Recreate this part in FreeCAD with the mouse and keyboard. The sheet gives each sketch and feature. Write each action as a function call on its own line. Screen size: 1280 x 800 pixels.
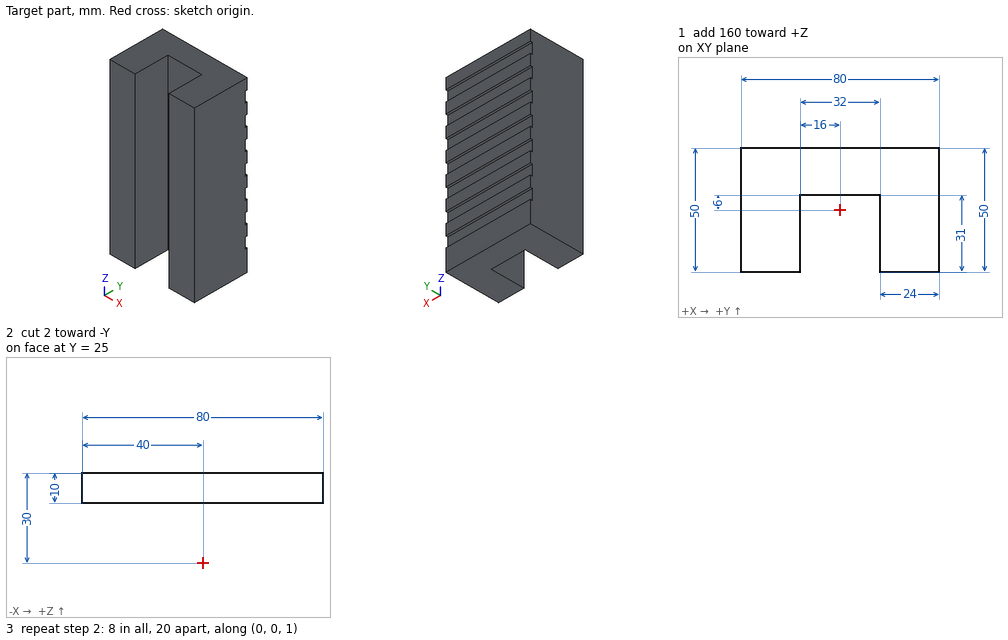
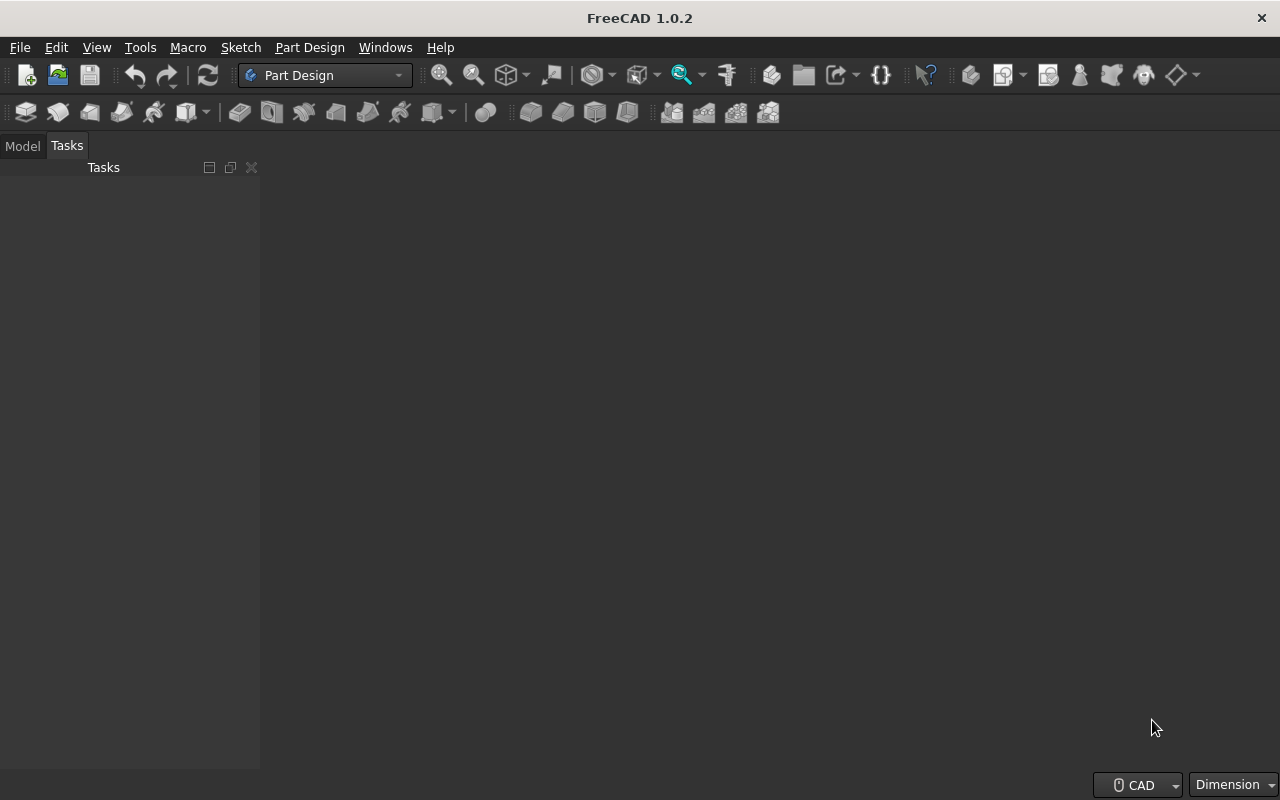
click(26, 76)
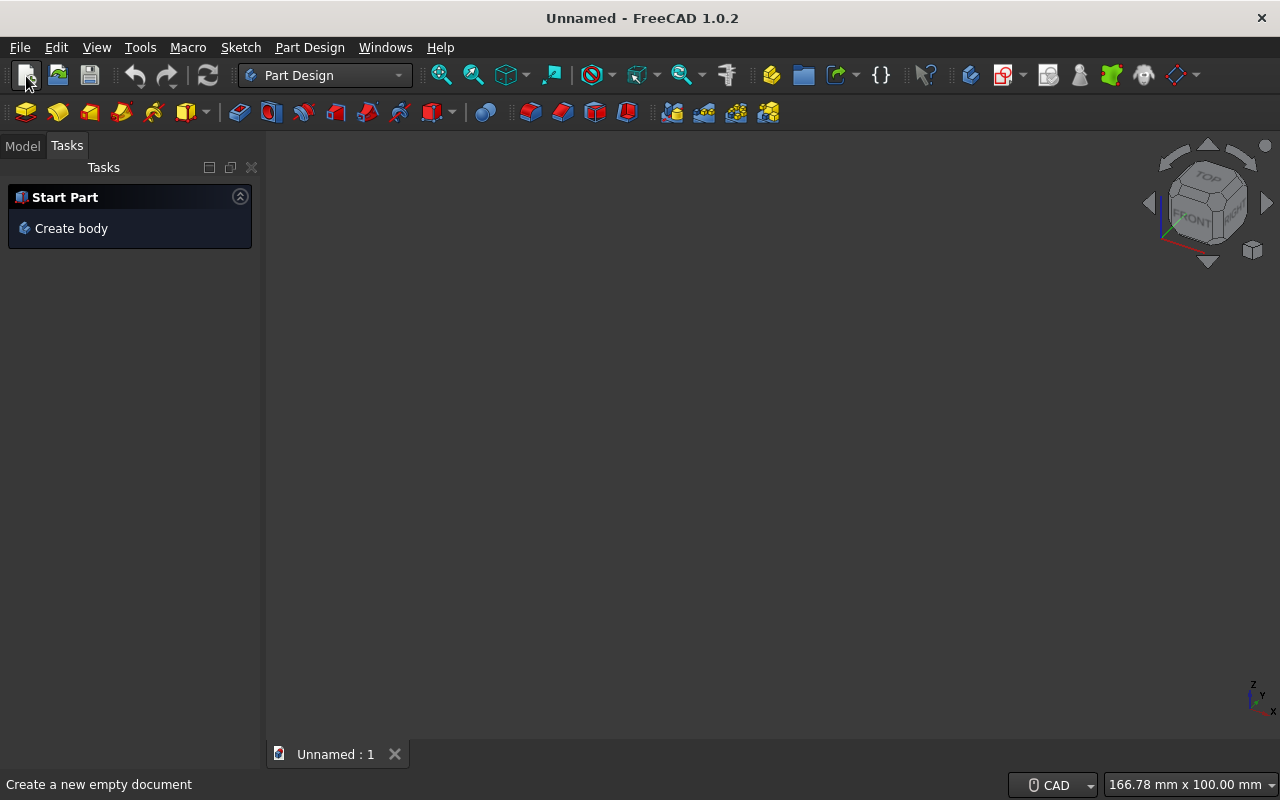
click(1004, 76)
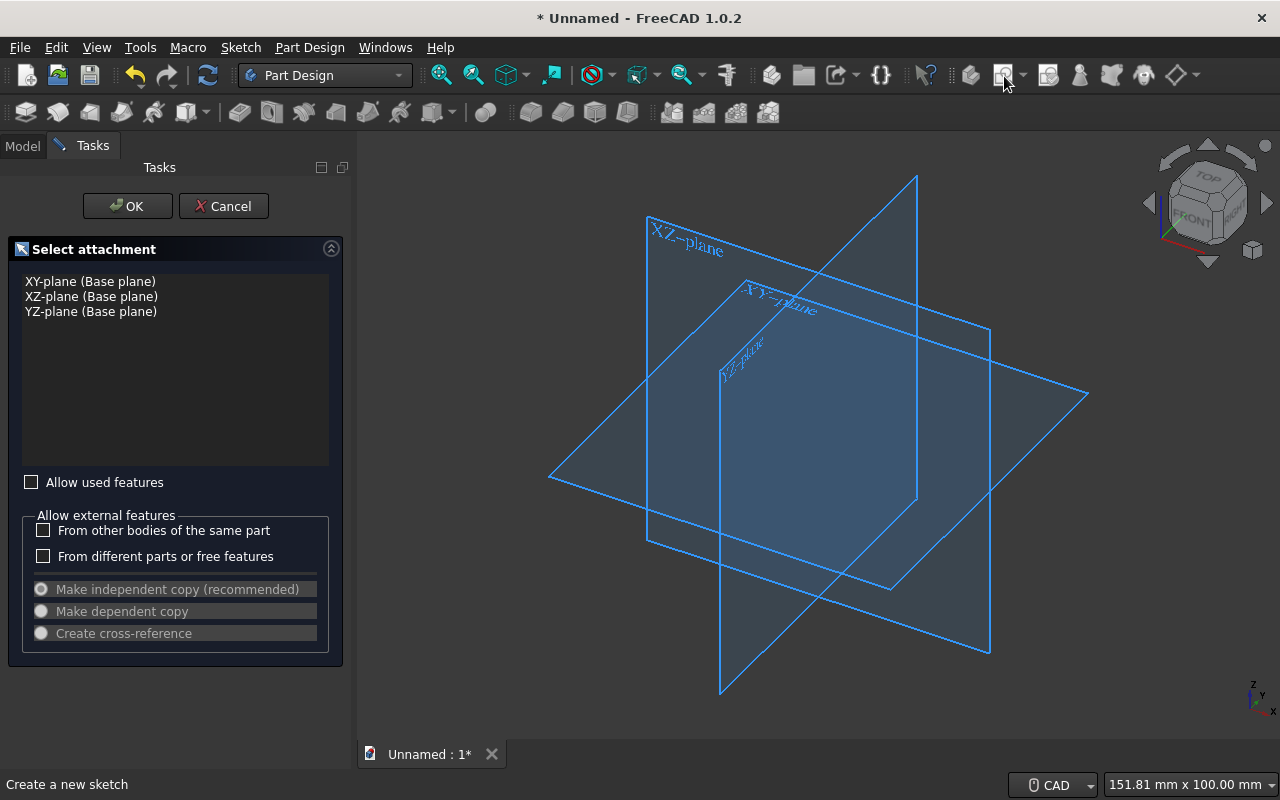
click(82, 282)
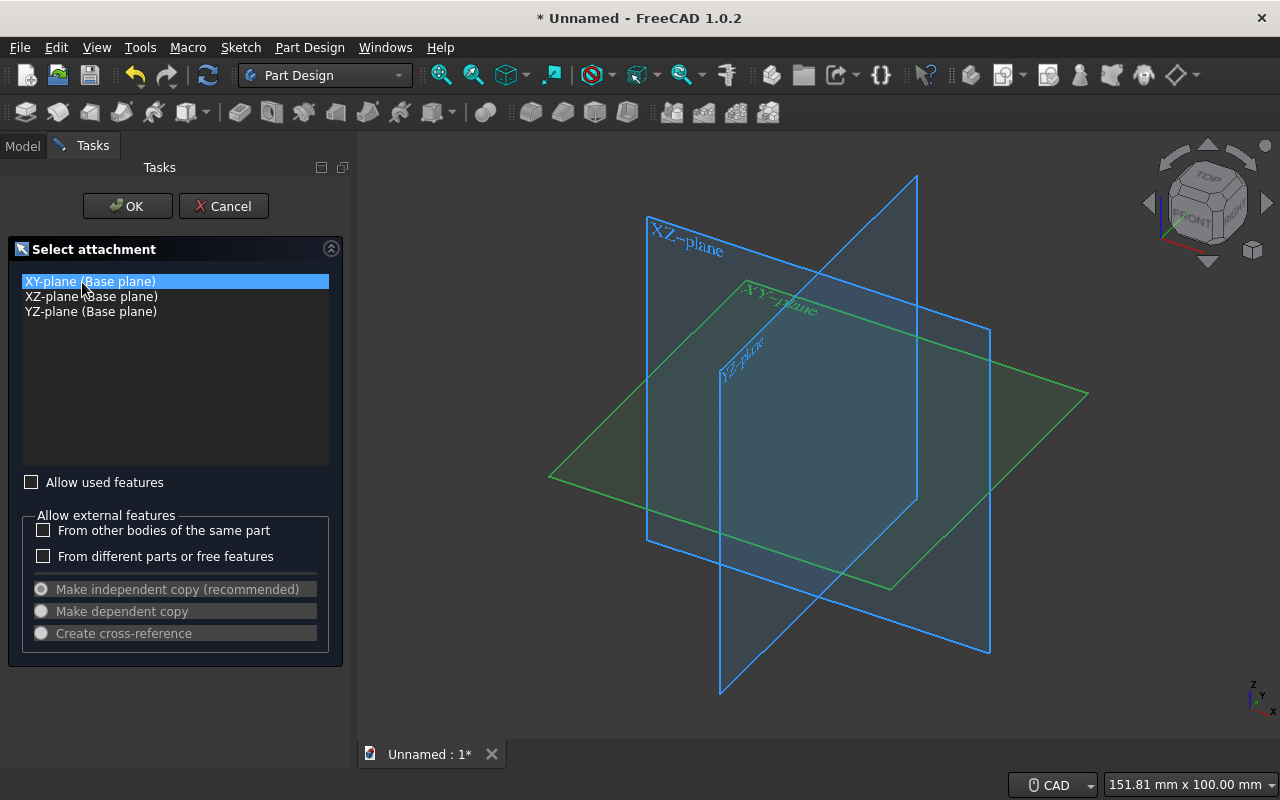
click(128, 206)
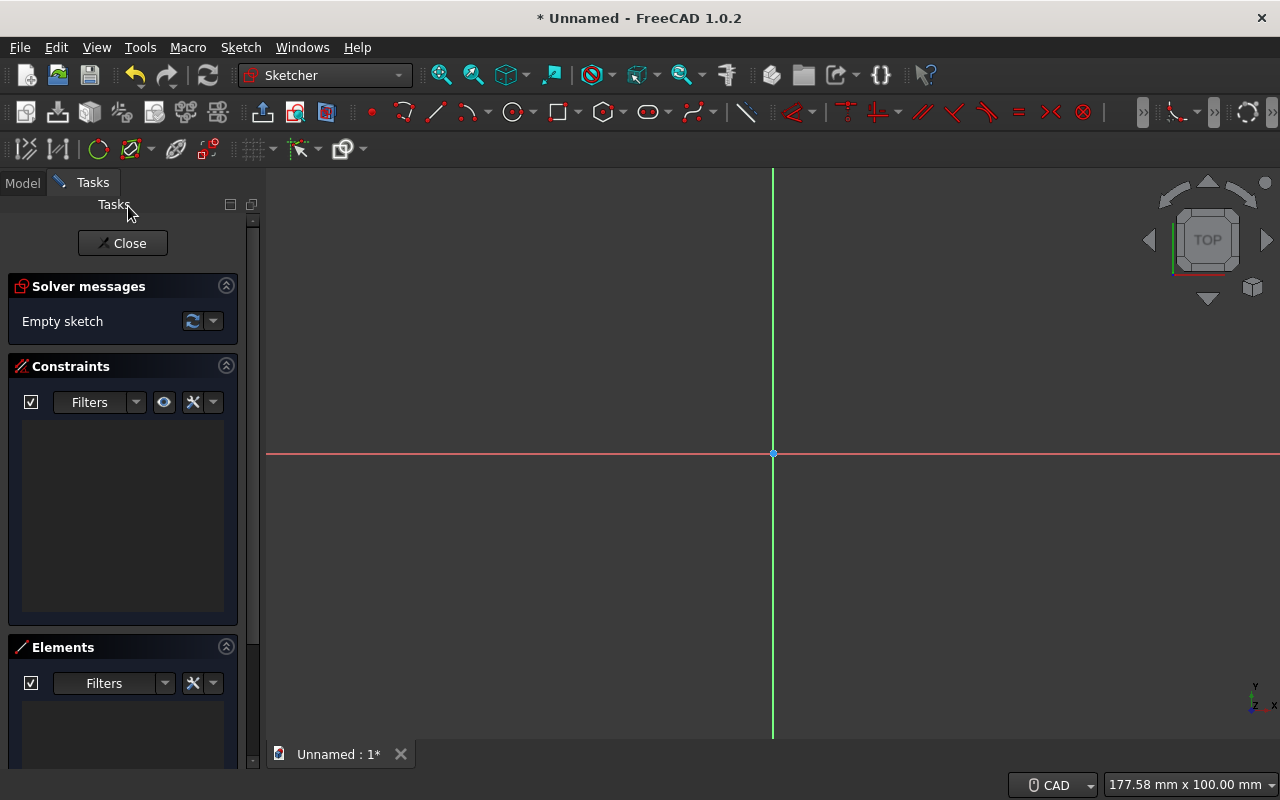
click(404, 112)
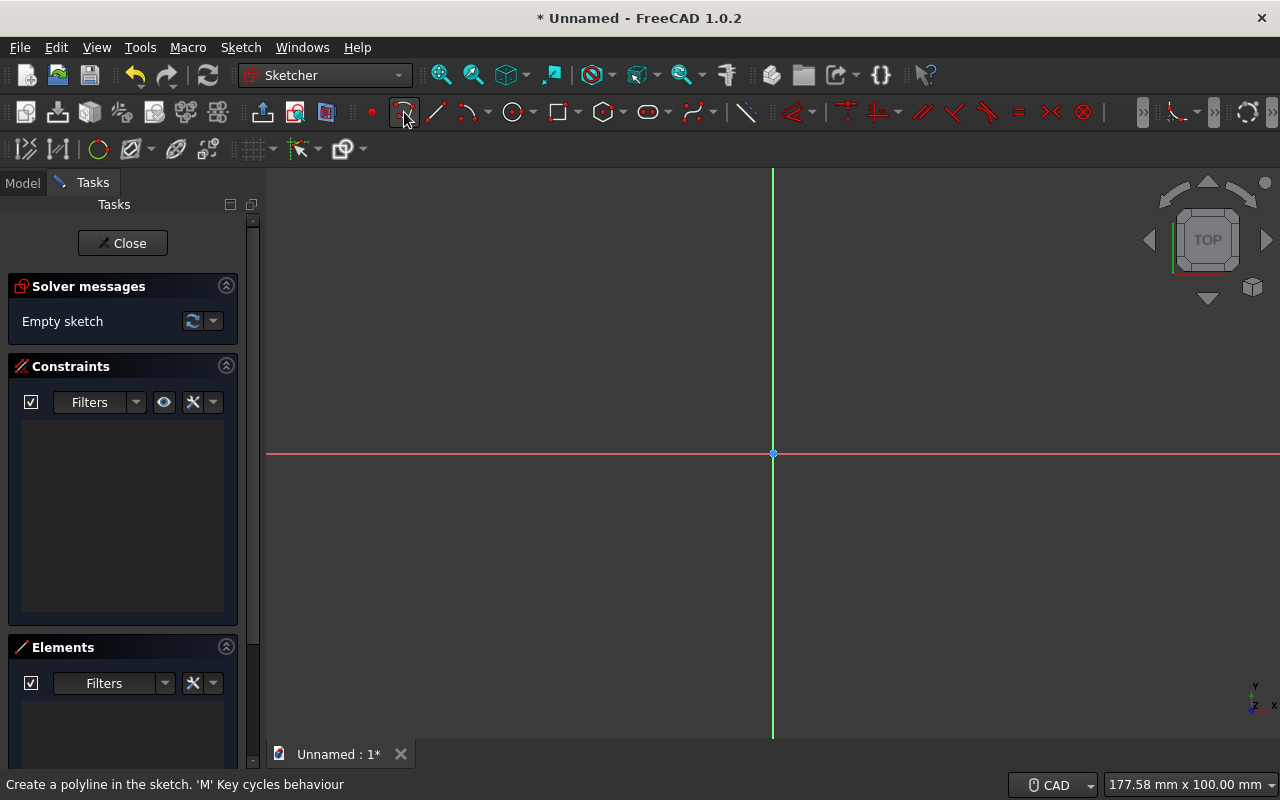
click(682, 419)
click(864, 419)
click(864, 596)
click(1001, 596)
click(1001, 311)
click(545, 311)
click(545, 596)
click(682, 596)
click(682, 420)
key(Escape)
key(Escape)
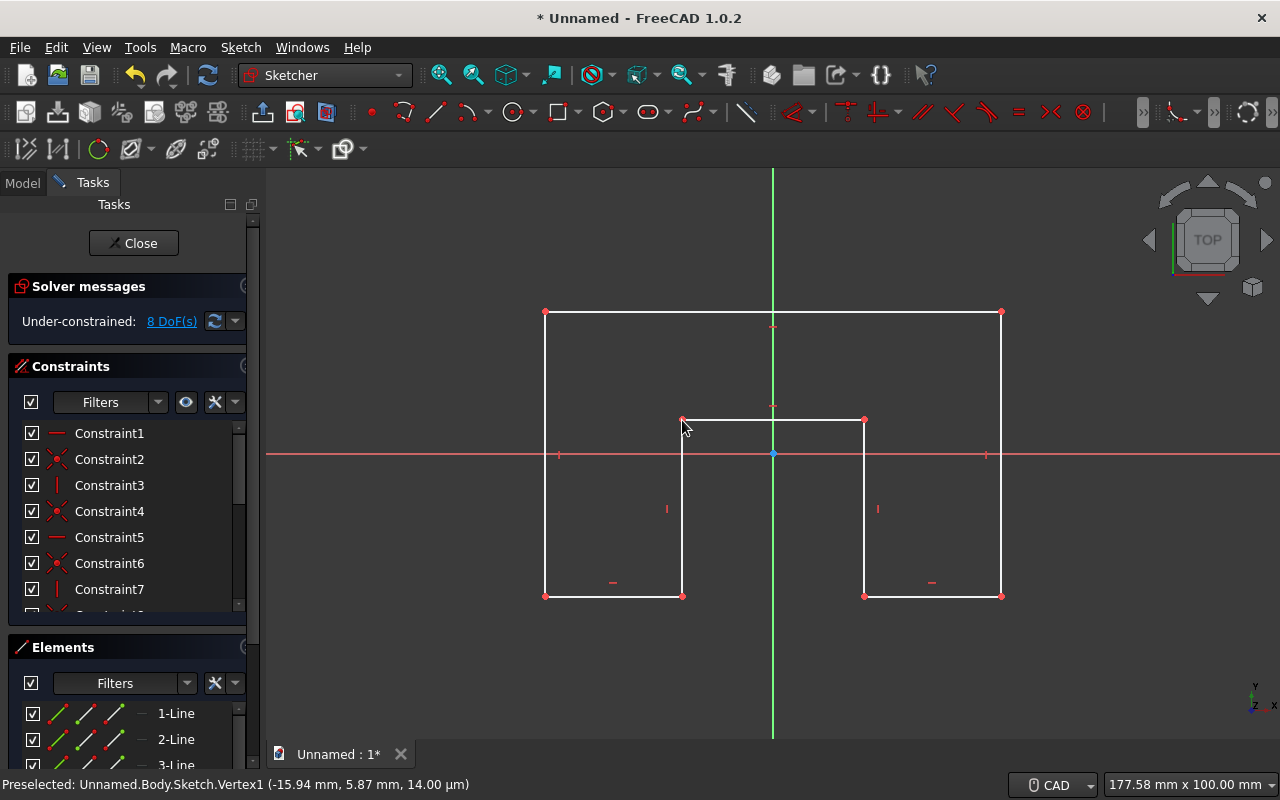
click(792, 112)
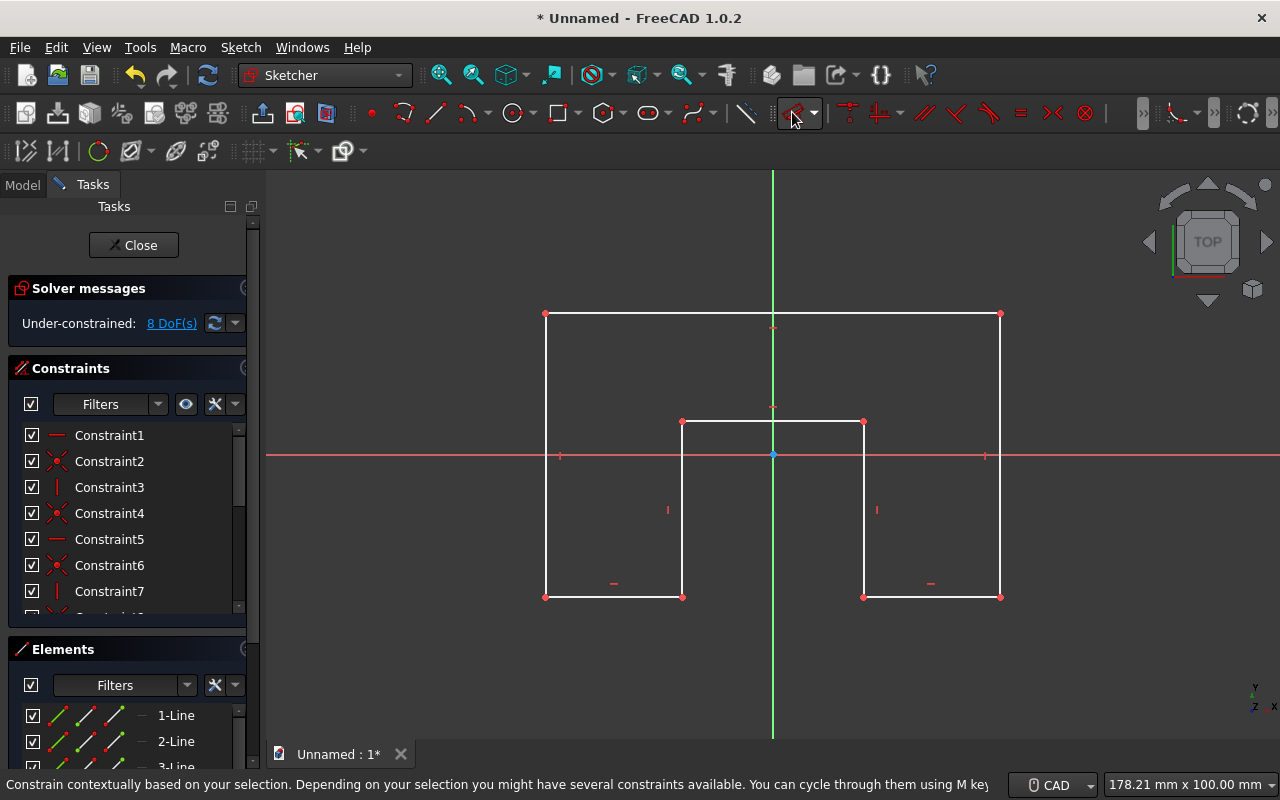
click(737, 421)
click(731, 387)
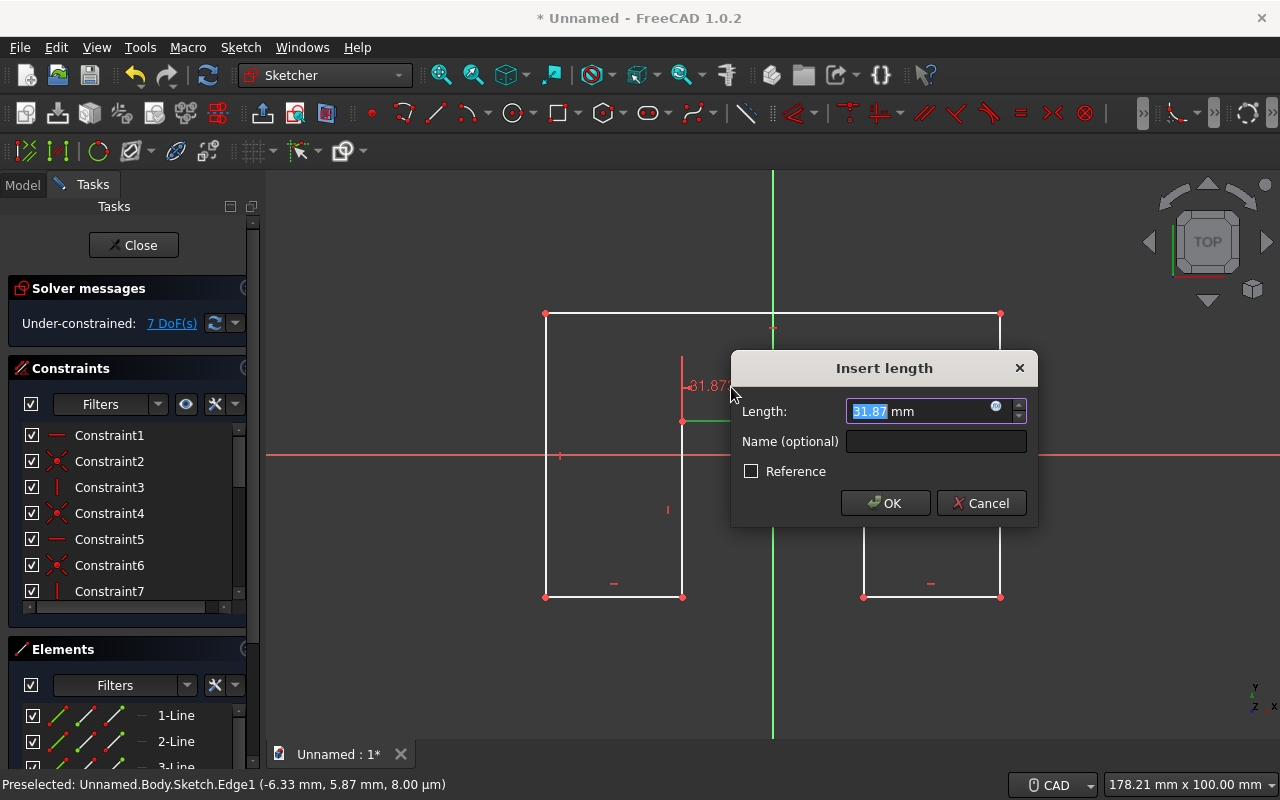
text(32)
key(Return)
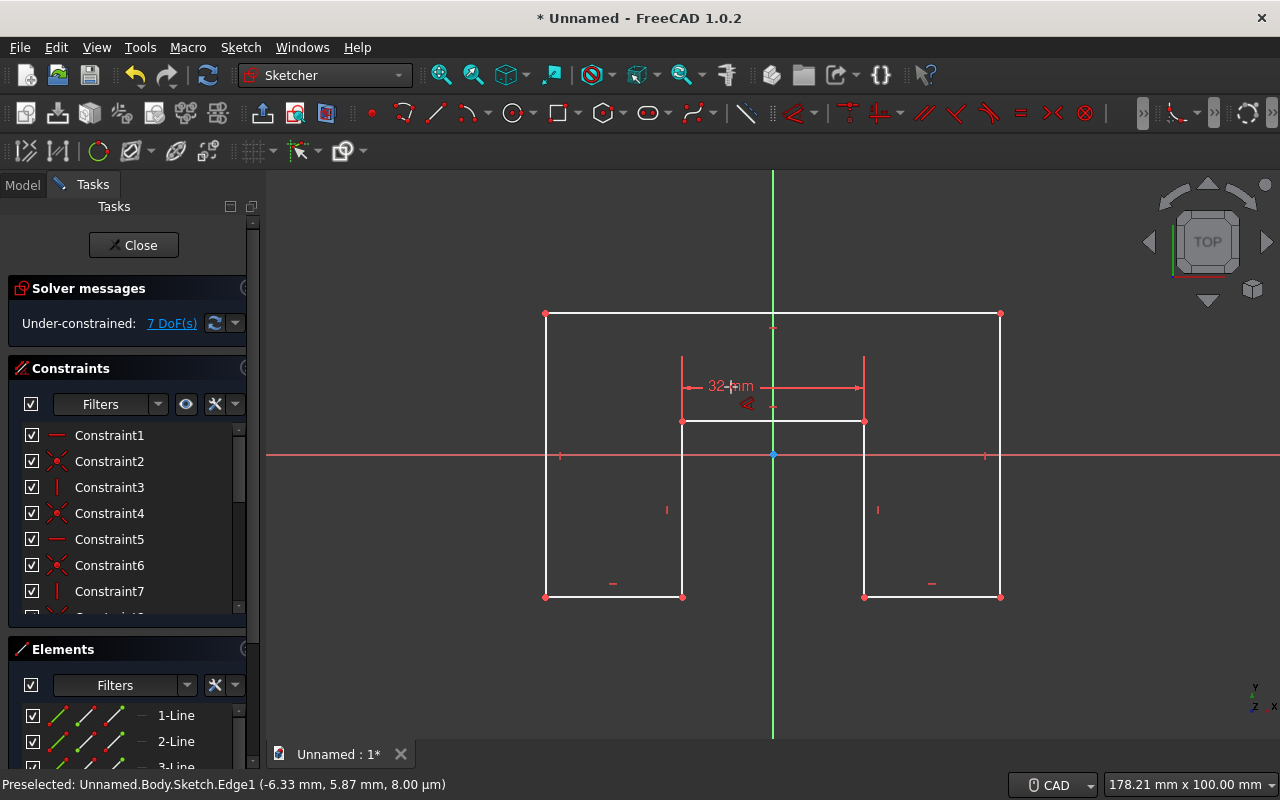
click(864, 474)
click(898, 509)